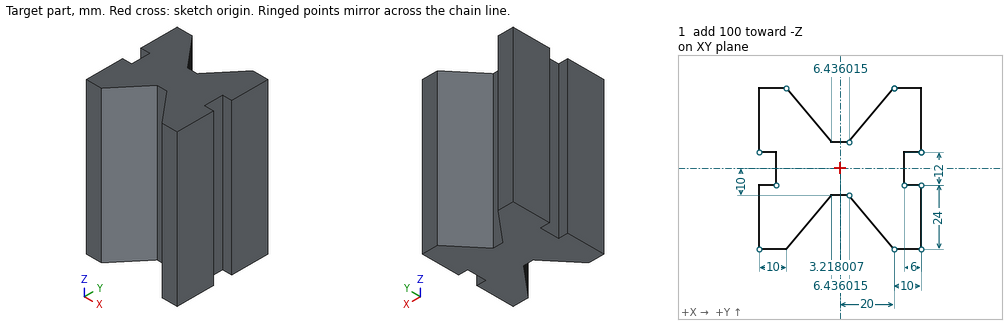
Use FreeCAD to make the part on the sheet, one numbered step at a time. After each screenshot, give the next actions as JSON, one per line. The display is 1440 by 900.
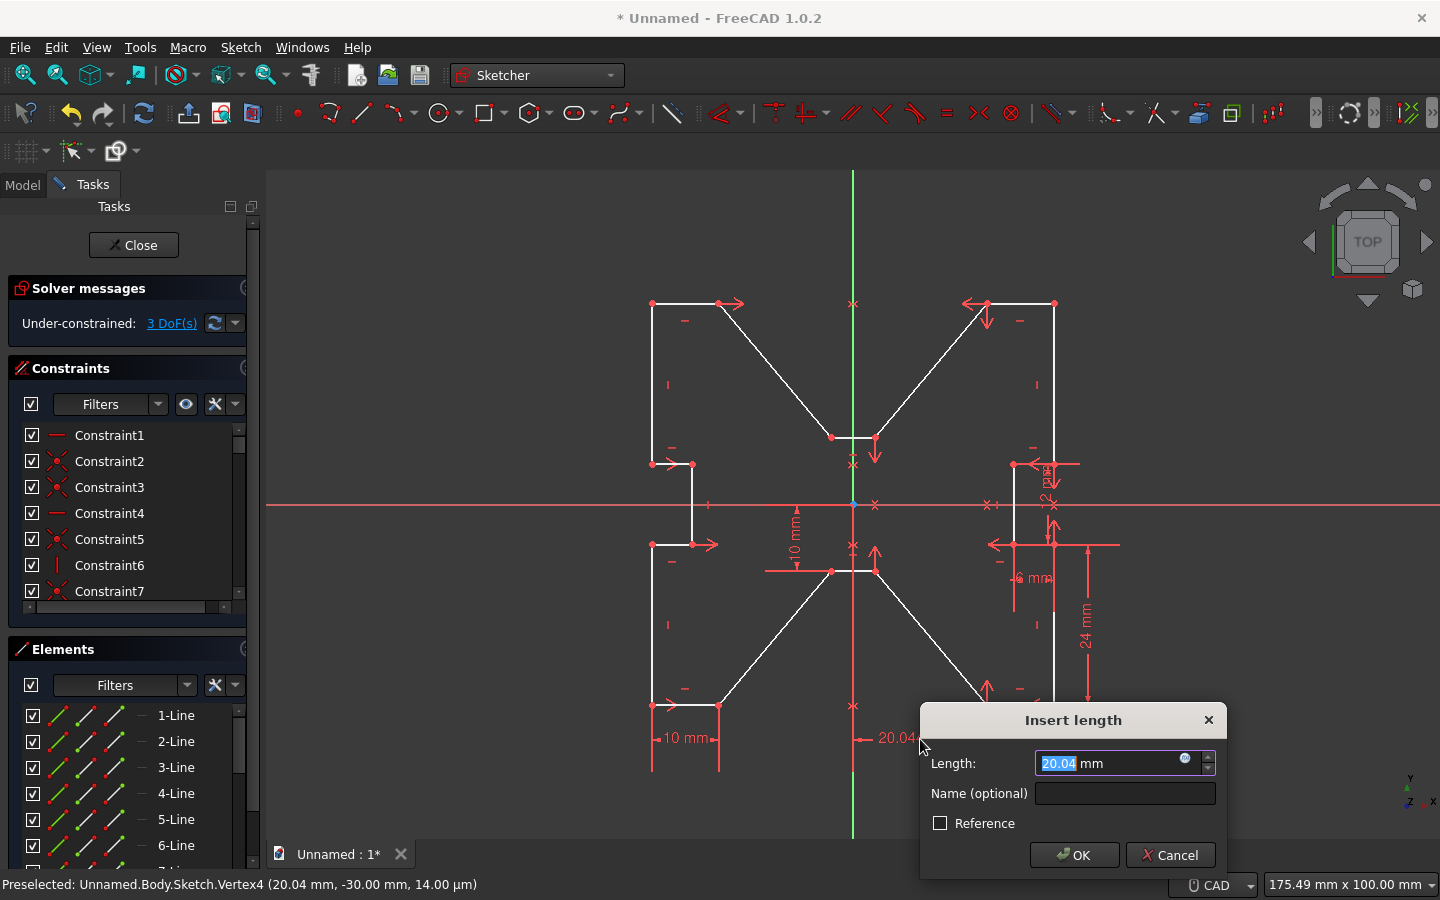
{"action": "type", "text": "20"}
{"action": "key", "text": "Return"}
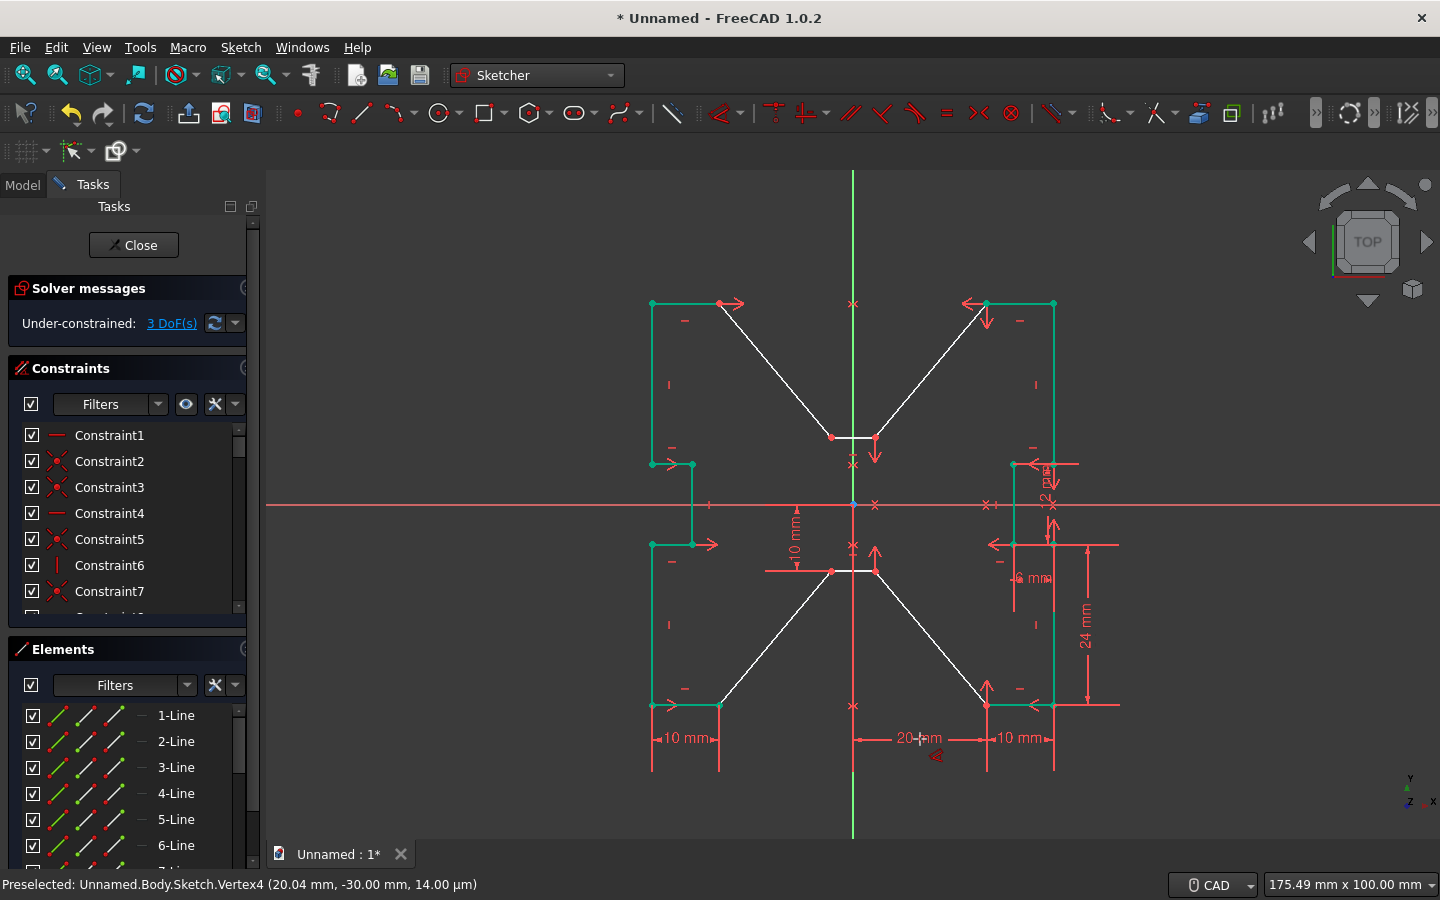
{"action": "left_click", "coordinate": [853, 571]}
{"action": "left_click", "coordinate": [838, 605]}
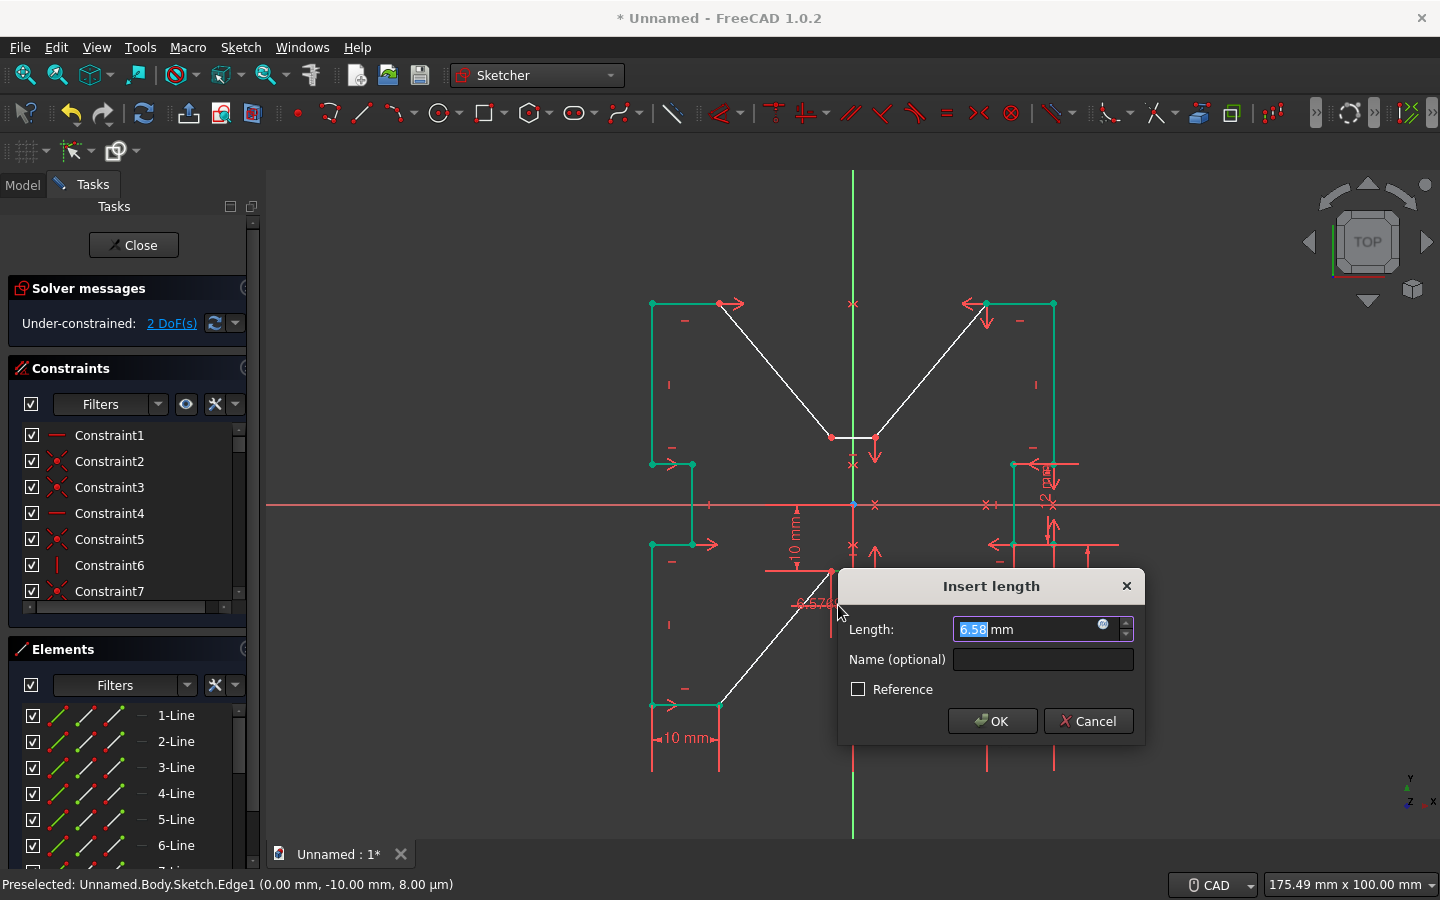
{"action": "type", "text": "6.436015"}
{"action": "key", "text": "Return"}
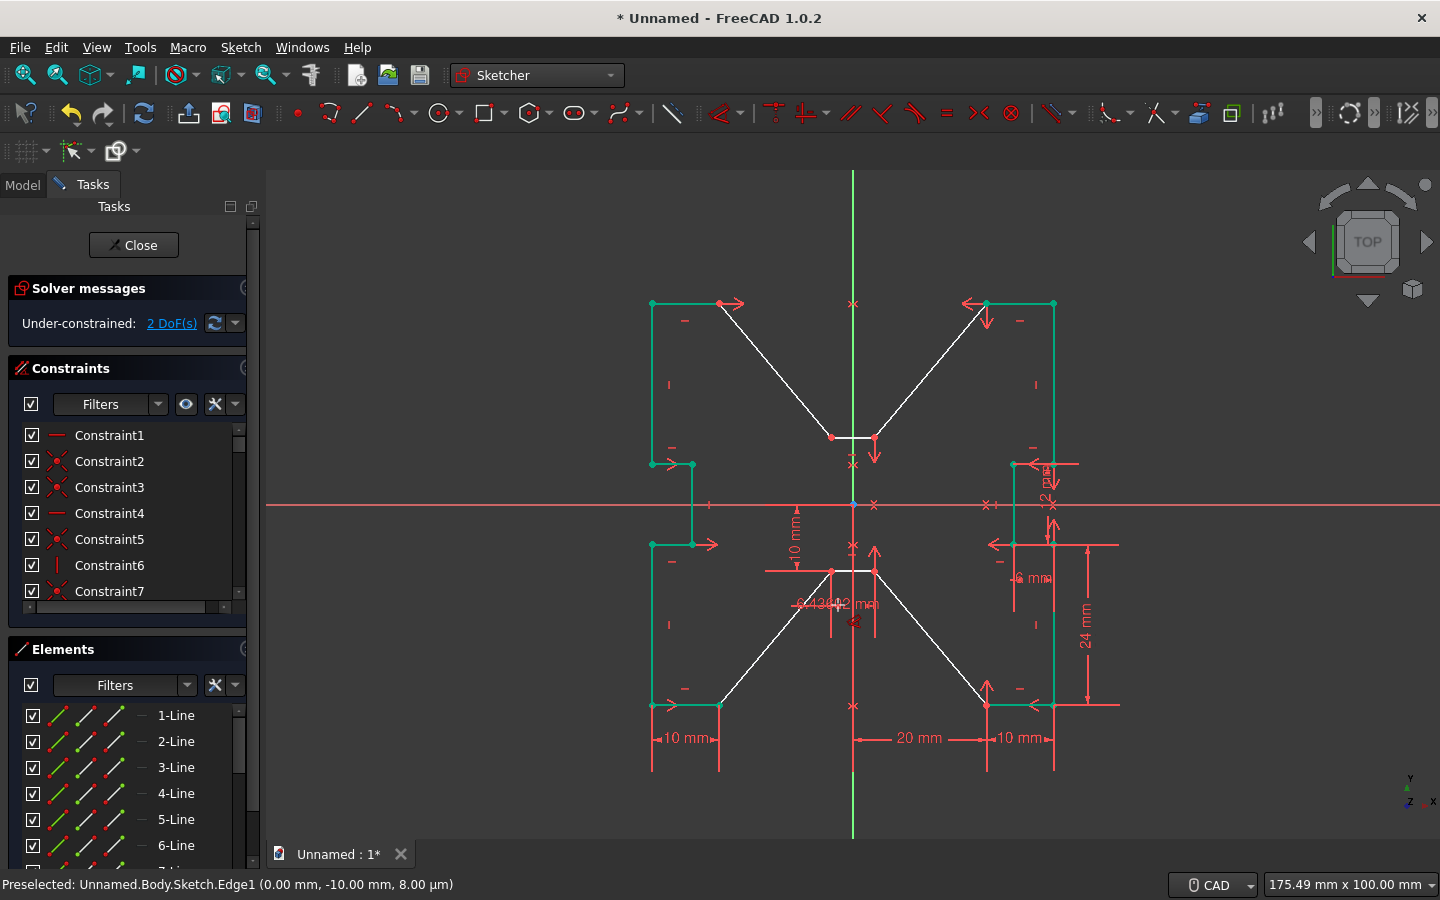
{"action": "left_click", "coordinate": [853, 438]}
{"action": "left_click", "coordinate": [838, 404]}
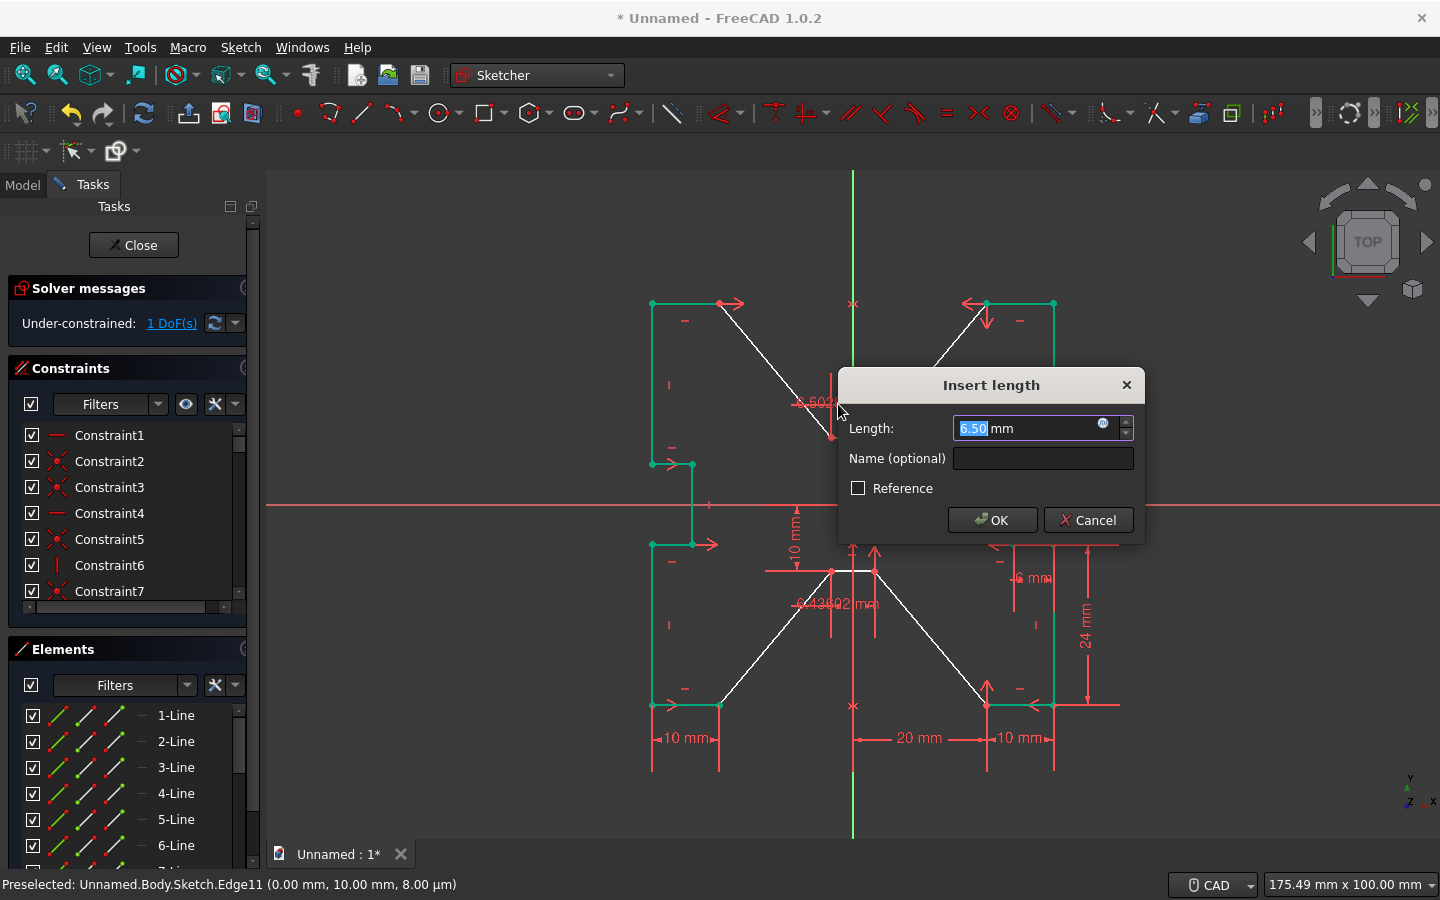
{"action": "type", "text": "6.436015"}
{"action": "key", "text": "Return"}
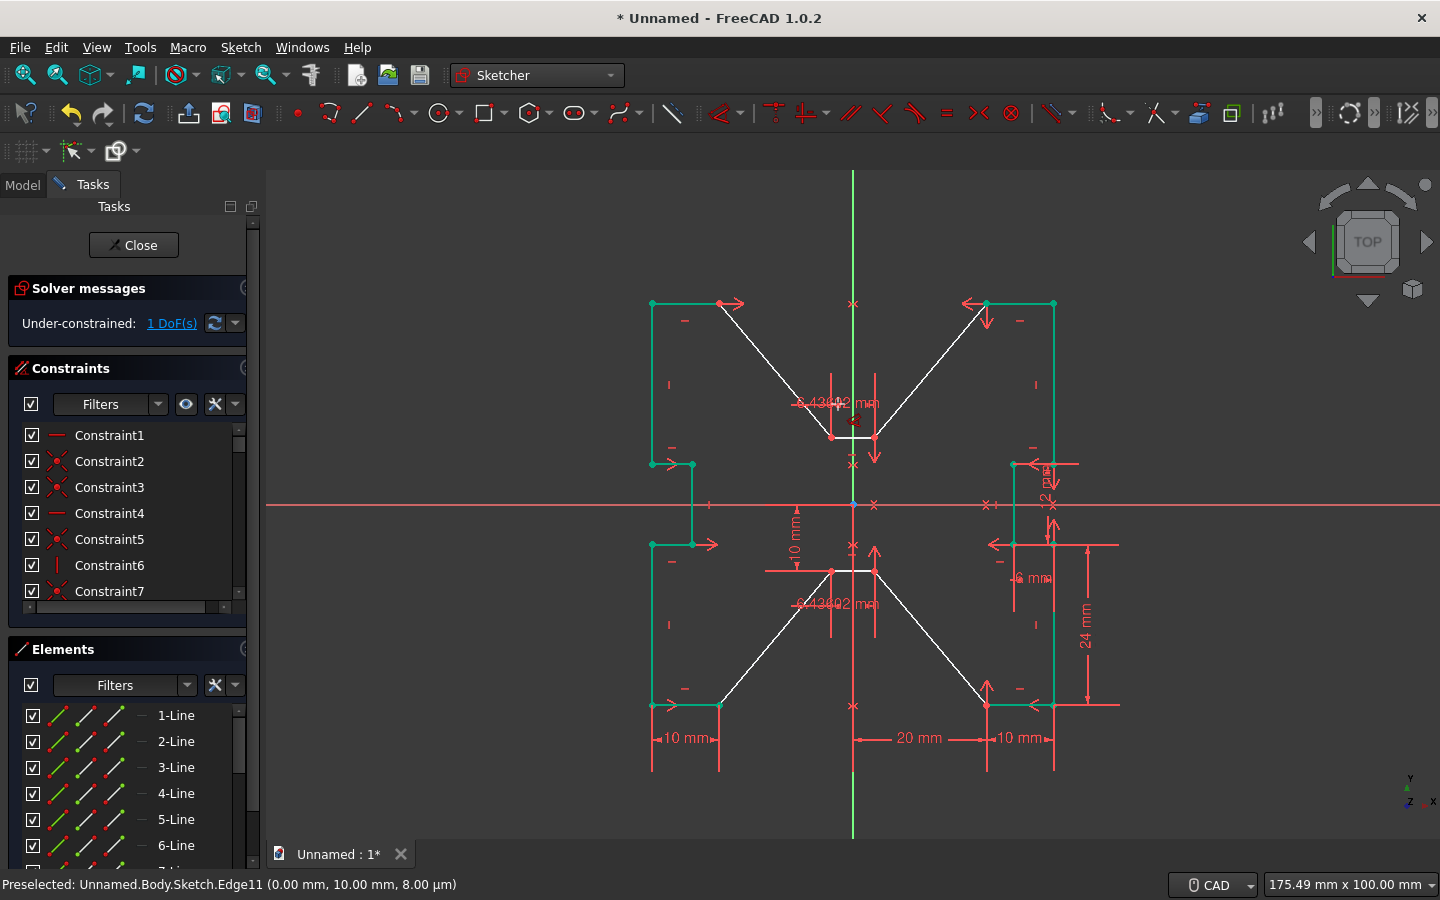
{"action": "scroll", "coordinate": [831, 571], "scroll_direction": "up", "scroll_amount": 4}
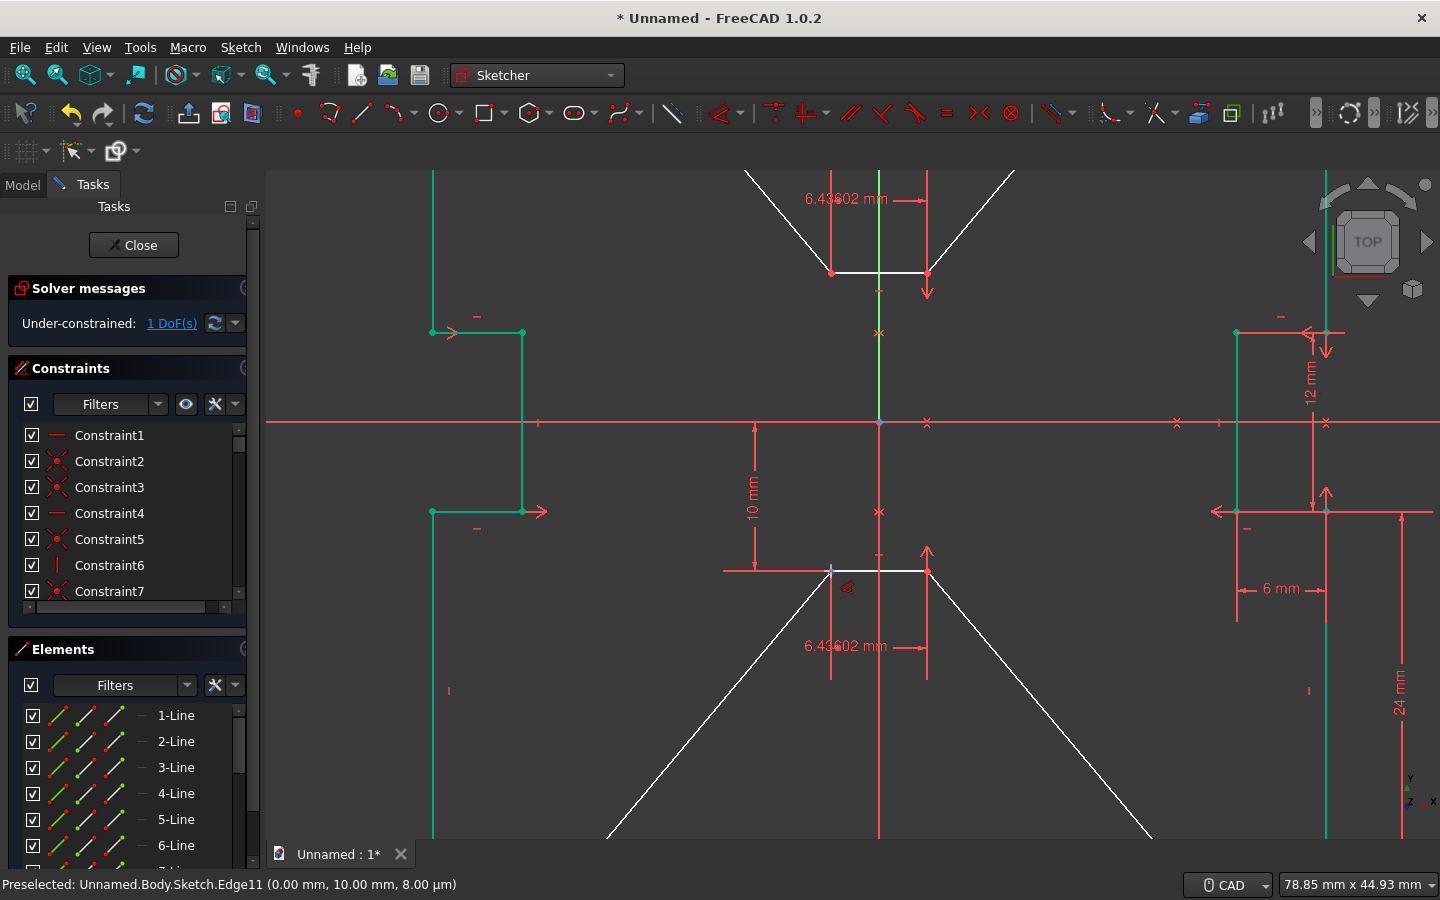
{"action": "left_click", "coordinate": [831, 571]}
{"action": "left_click", "coordinate": [855, 605]}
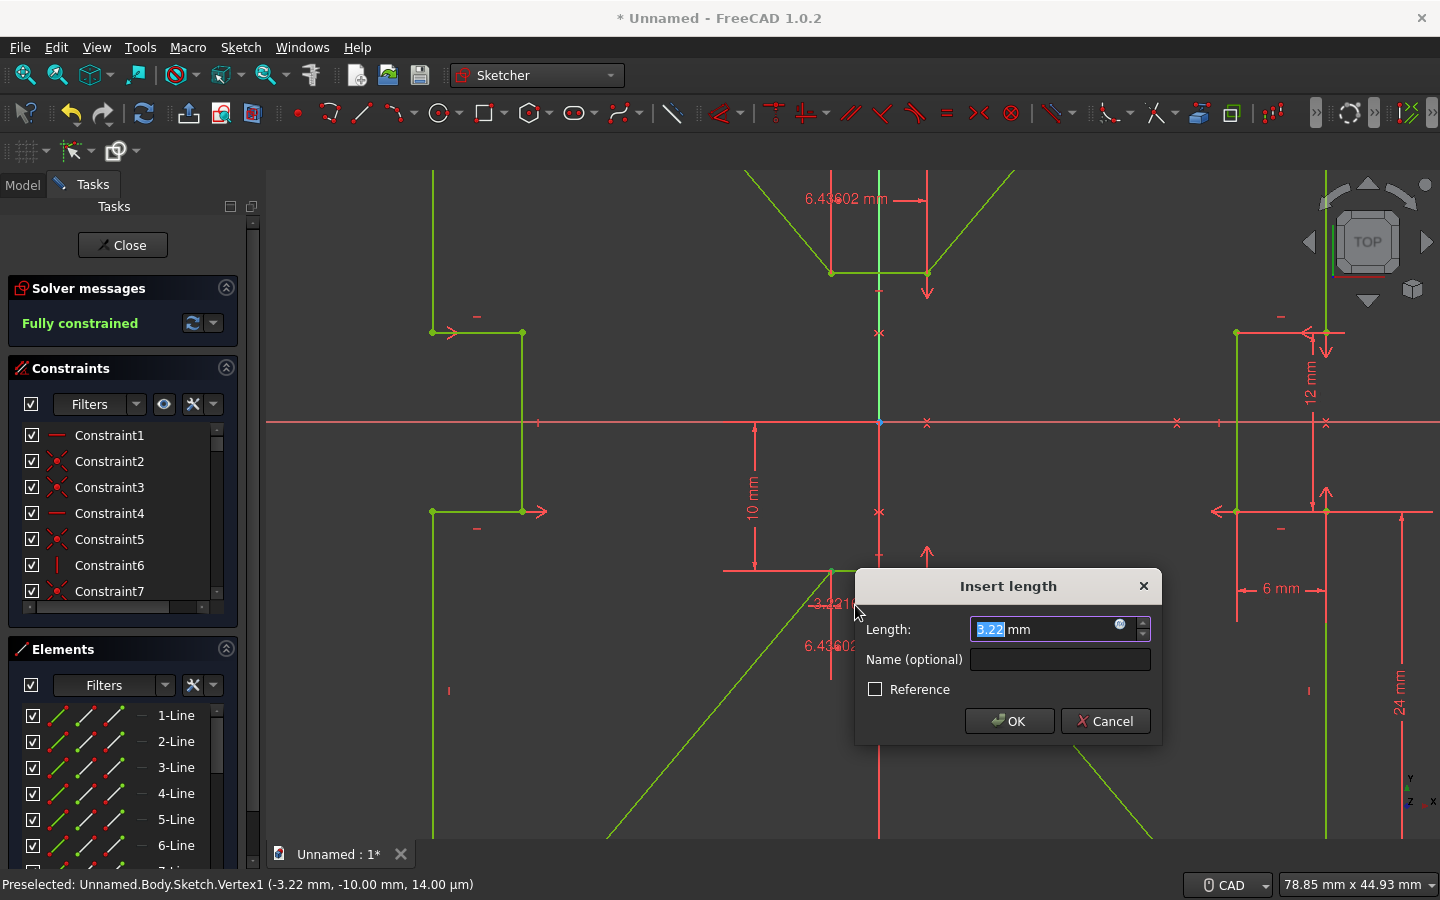
{"action": "type", "text": "3.218007"}
{"action": "key", "text": "Return"}
{"action": "key", "text": "Escape"}